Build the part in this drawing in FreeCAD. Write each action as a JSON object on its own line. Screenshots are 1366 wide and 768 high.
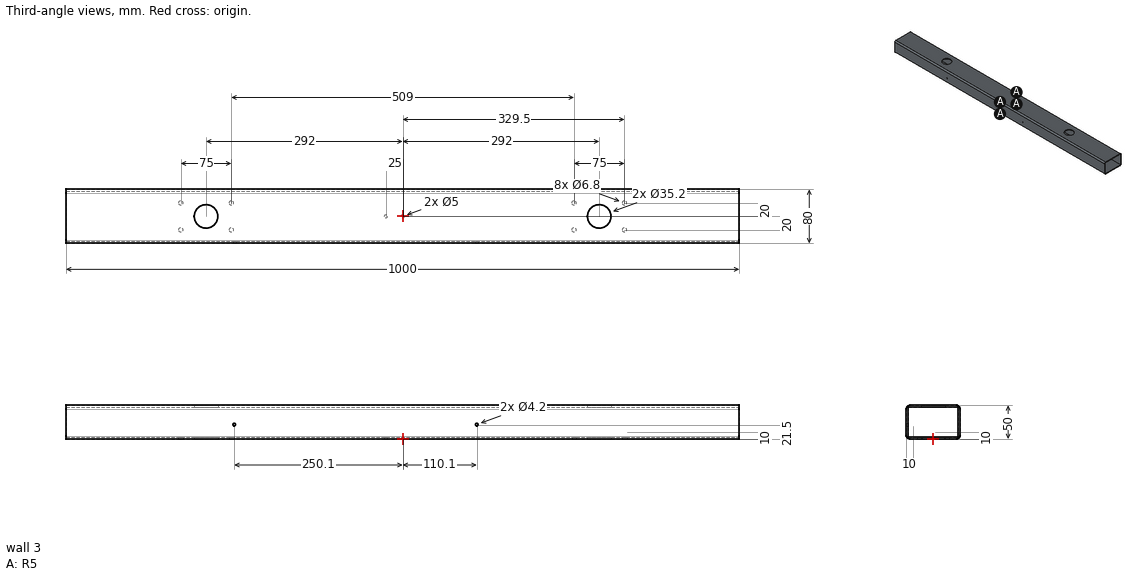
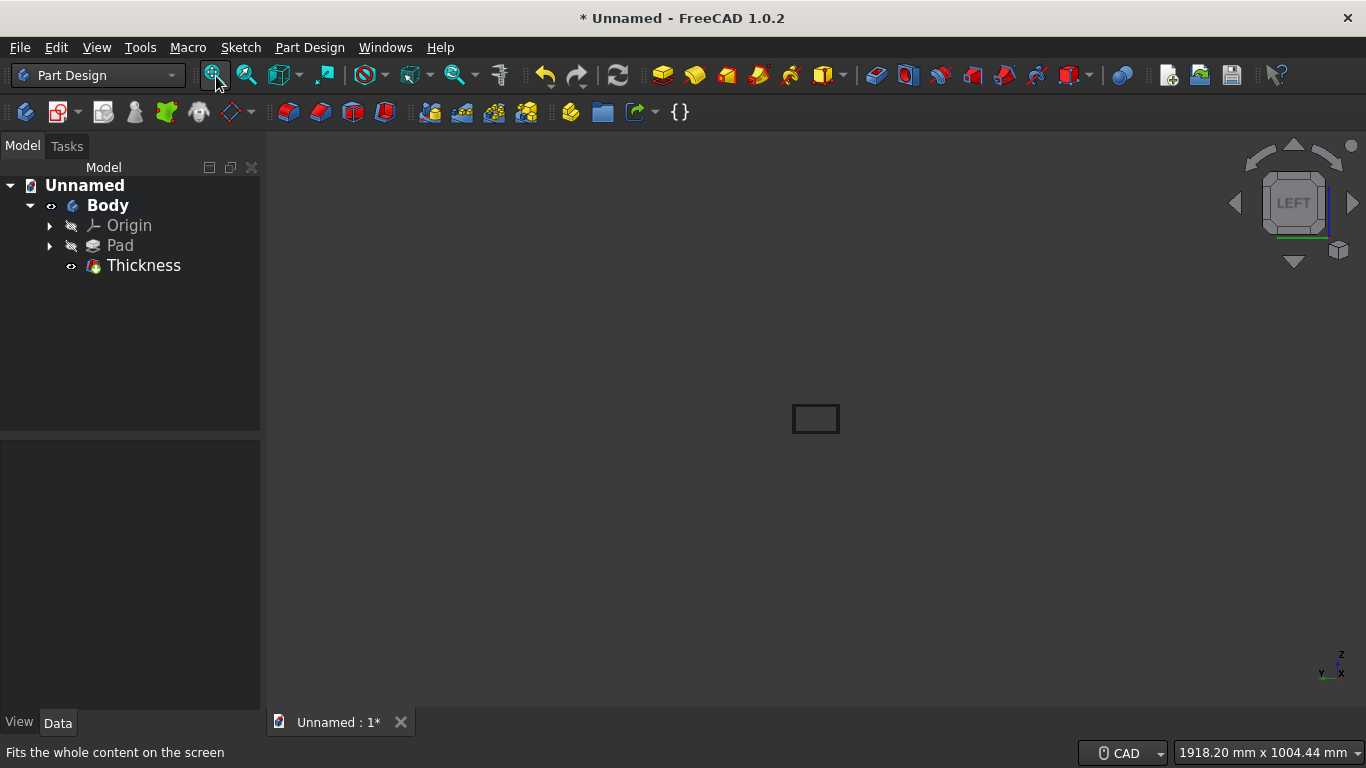
{"action": "key", "text": "0"}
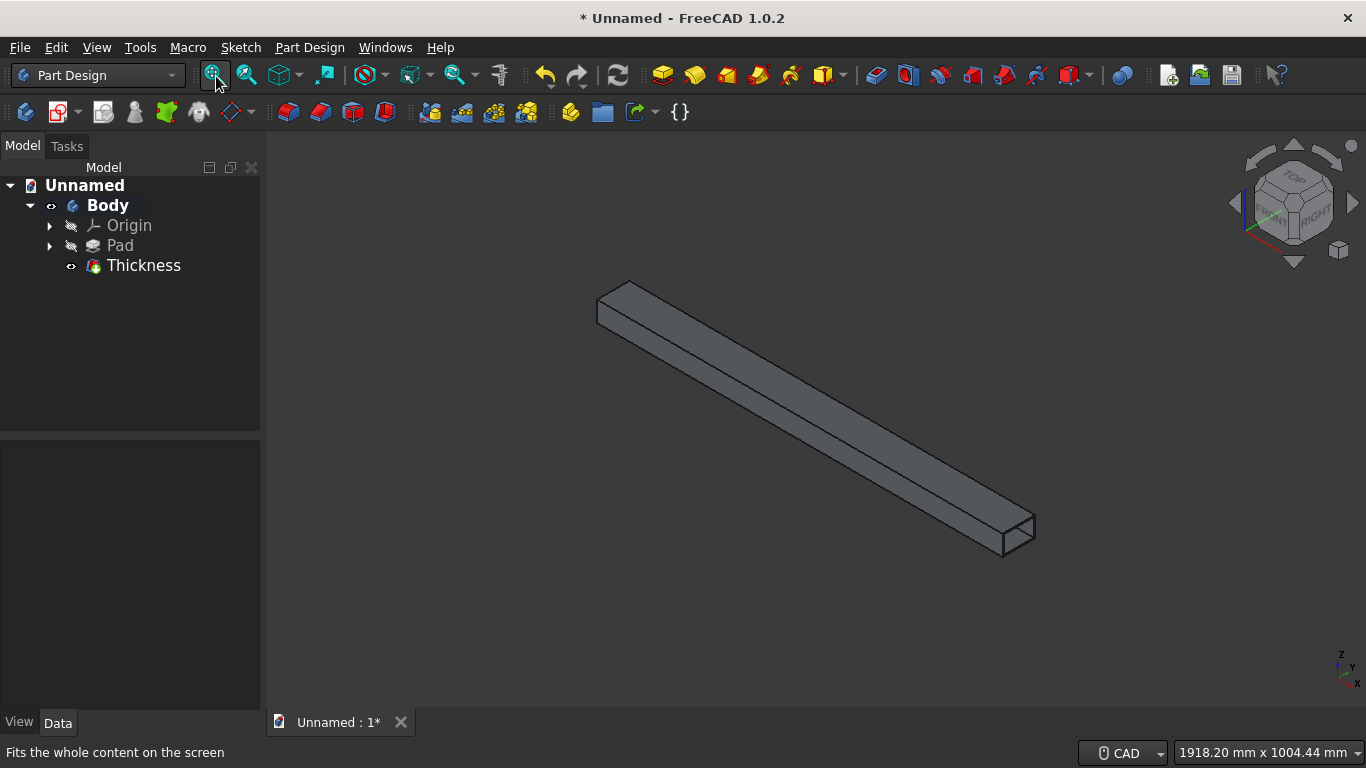
{"action": "left_click", "coordinate": [800, 416]}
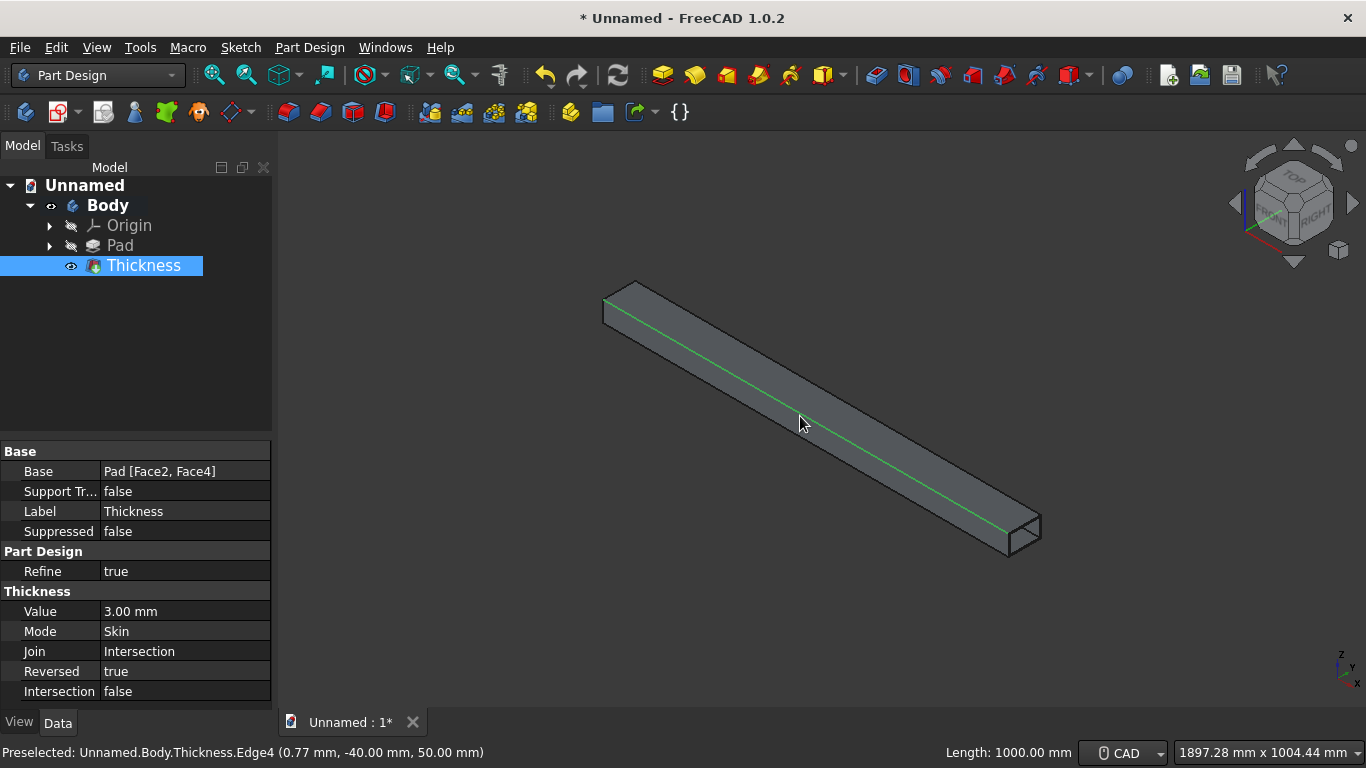
{"action": "key", "text": "2"}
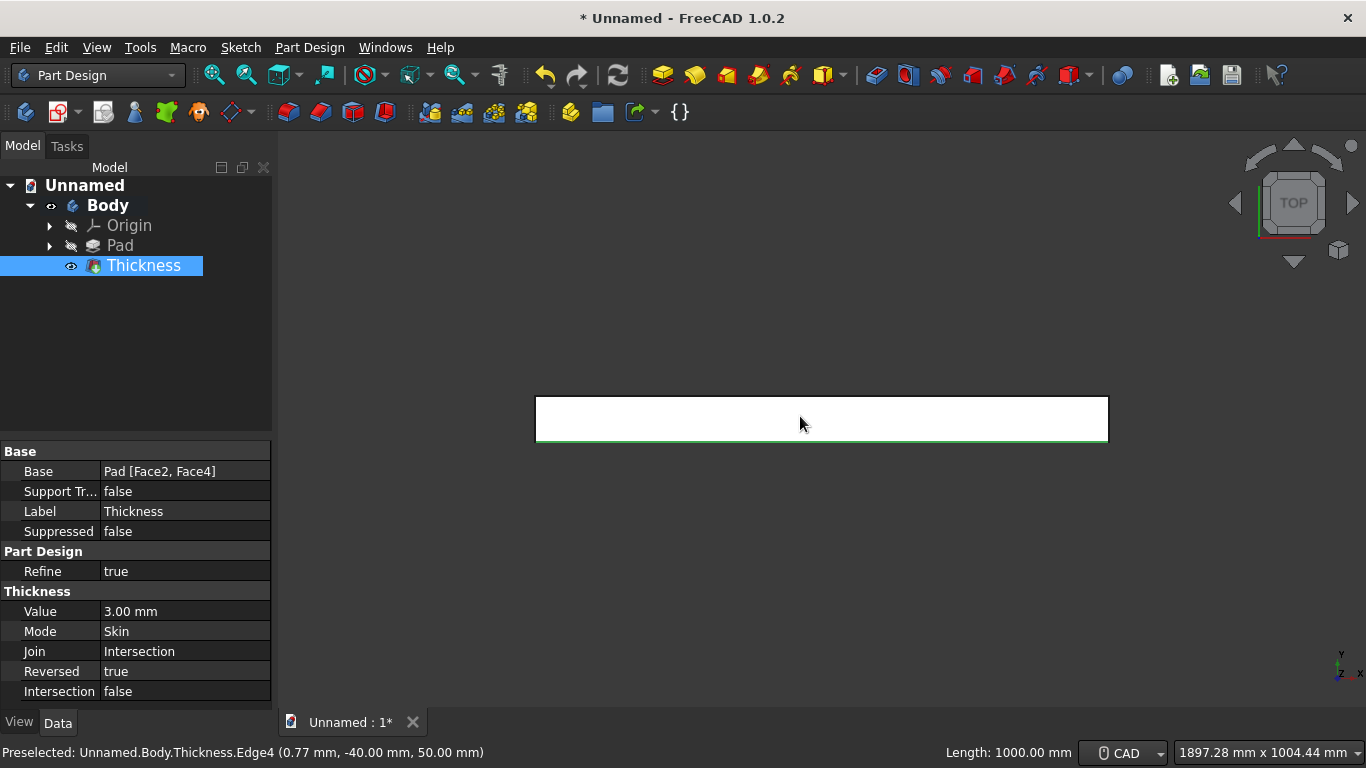
{"action": "left_click", "coordinate": [822, 395], "text": "ctrl"}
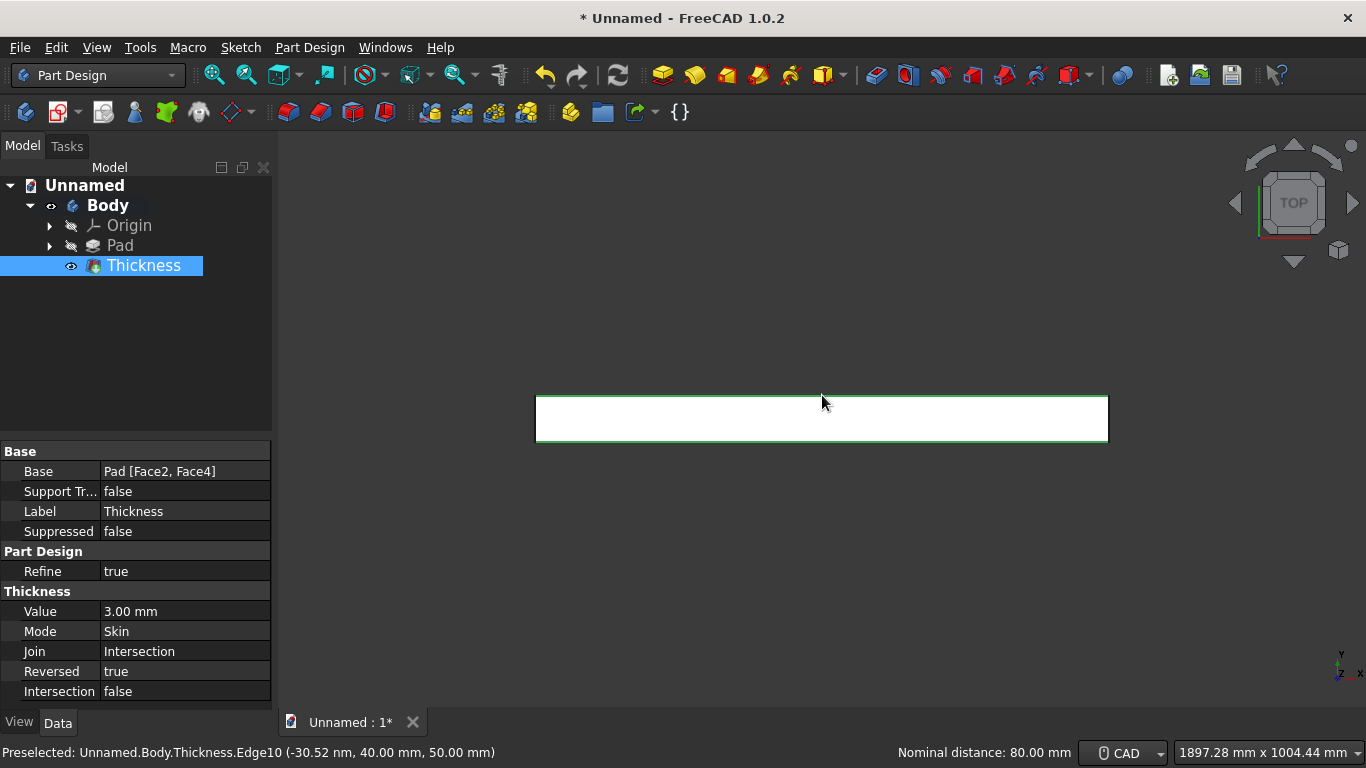
{"action": "key", "text": "1"}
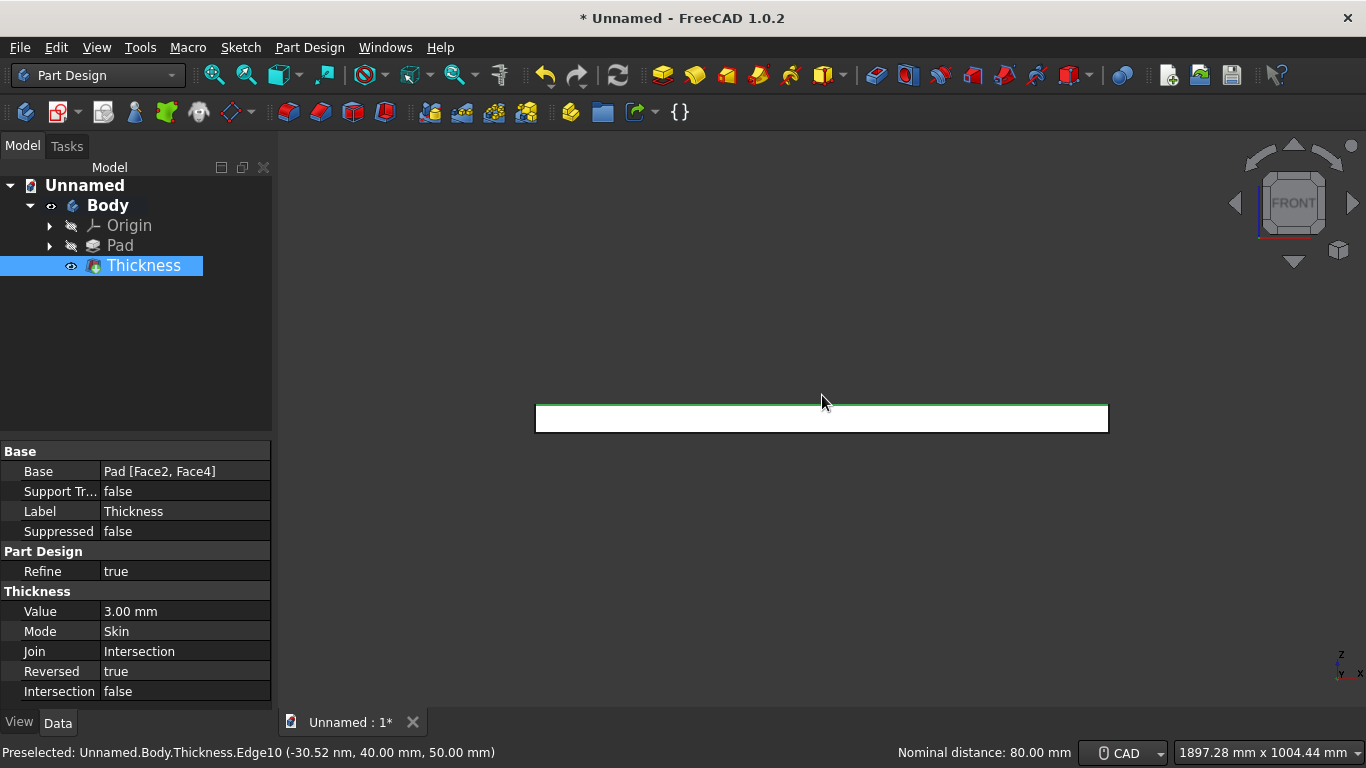
{"action": "left_click", "coordinate": [822, 432], "text": "ctrl"}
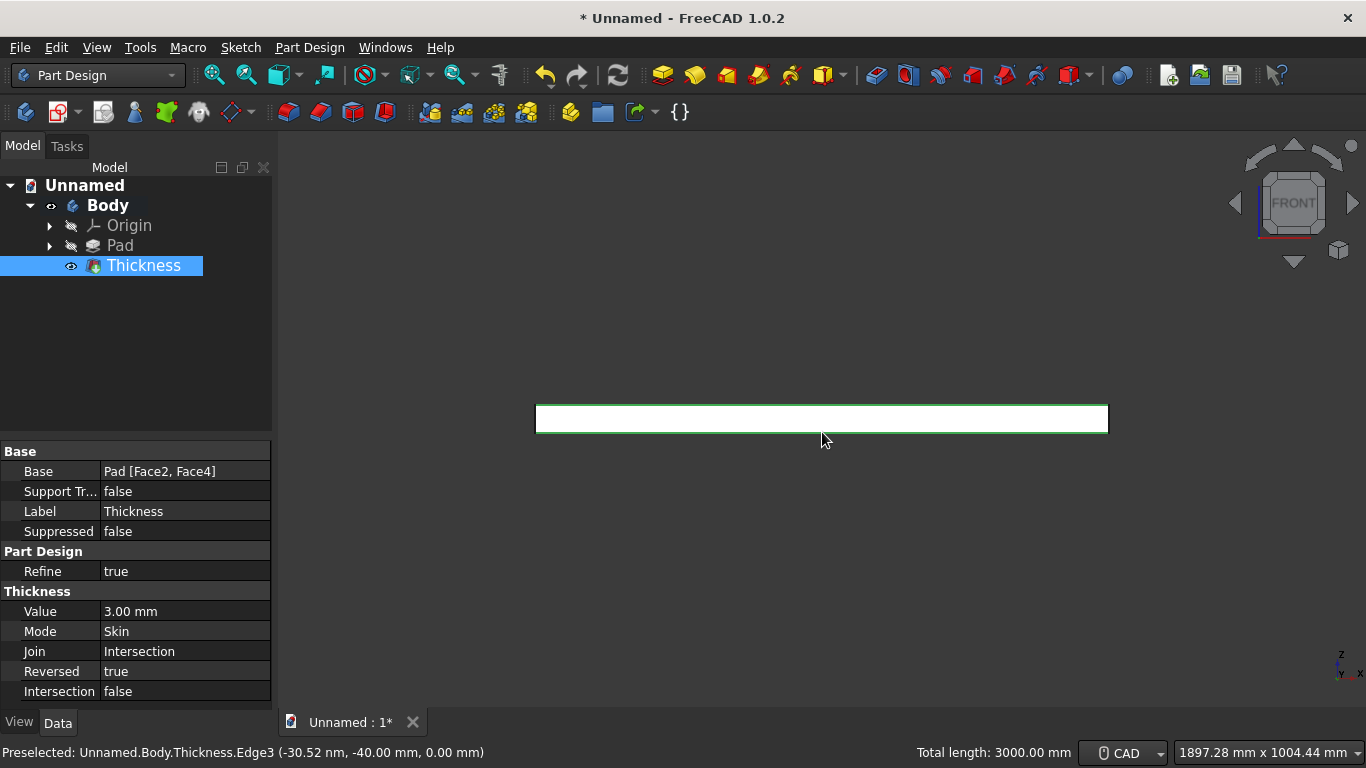
{"action": "key", "text": "3"}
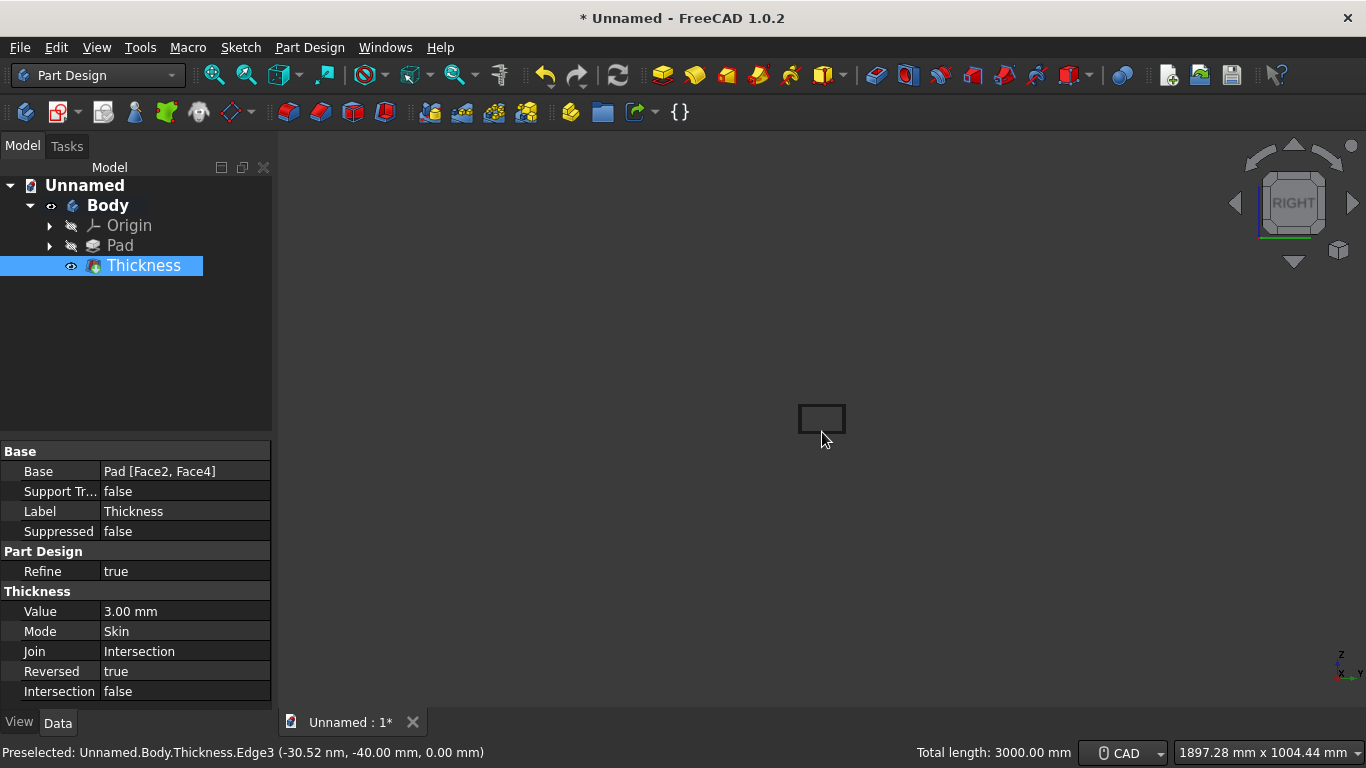
{"action": "left_click", "coordinate": [216, 76]}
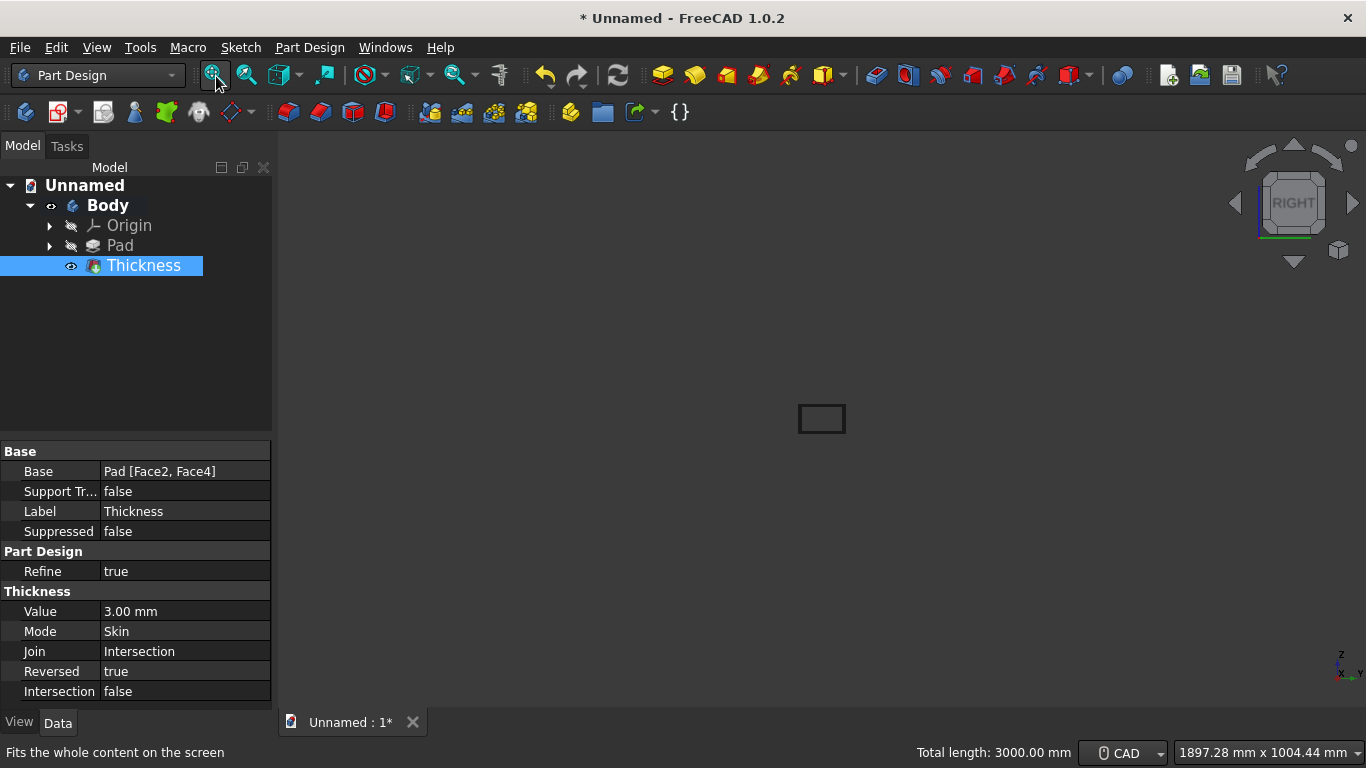
{"action": "key", "text": "5"}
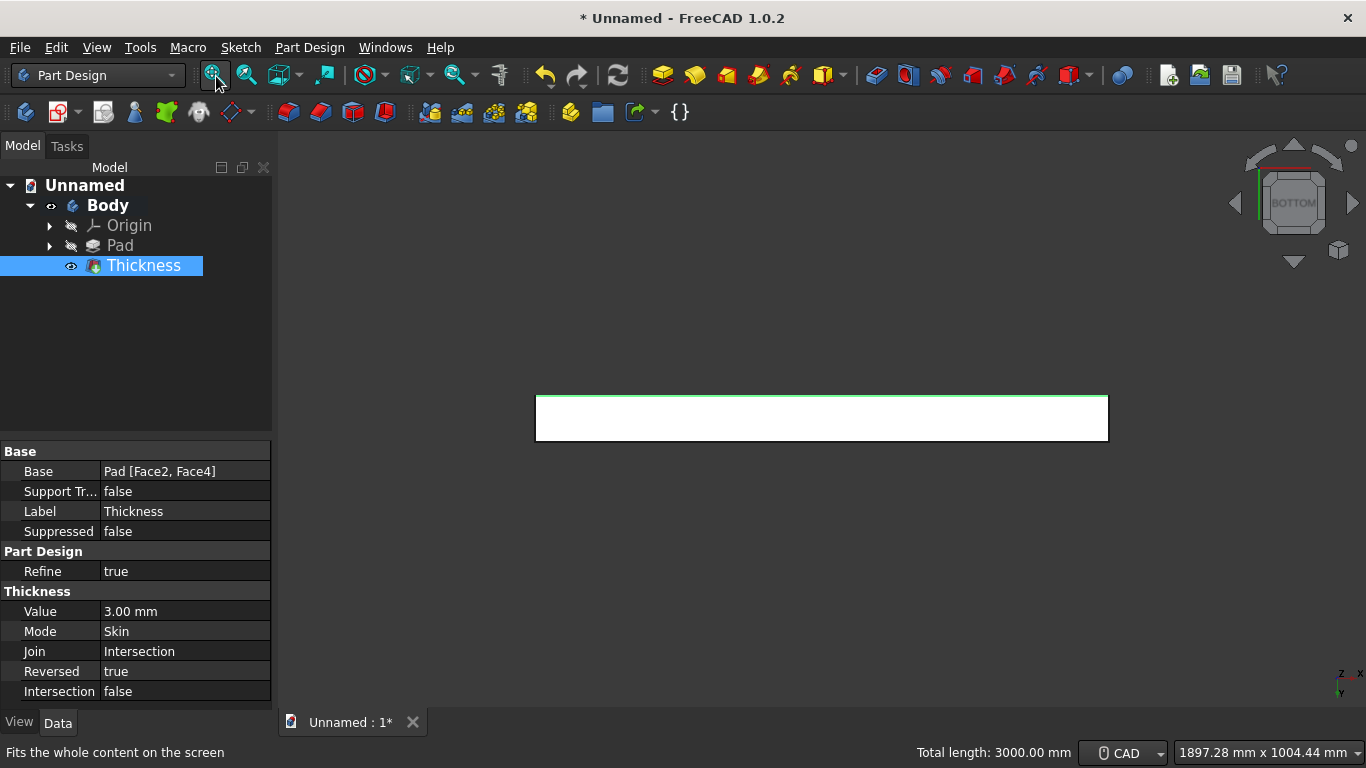
{"action": "left_click", "coordinate": [822, 441], "text": "ctrl"}